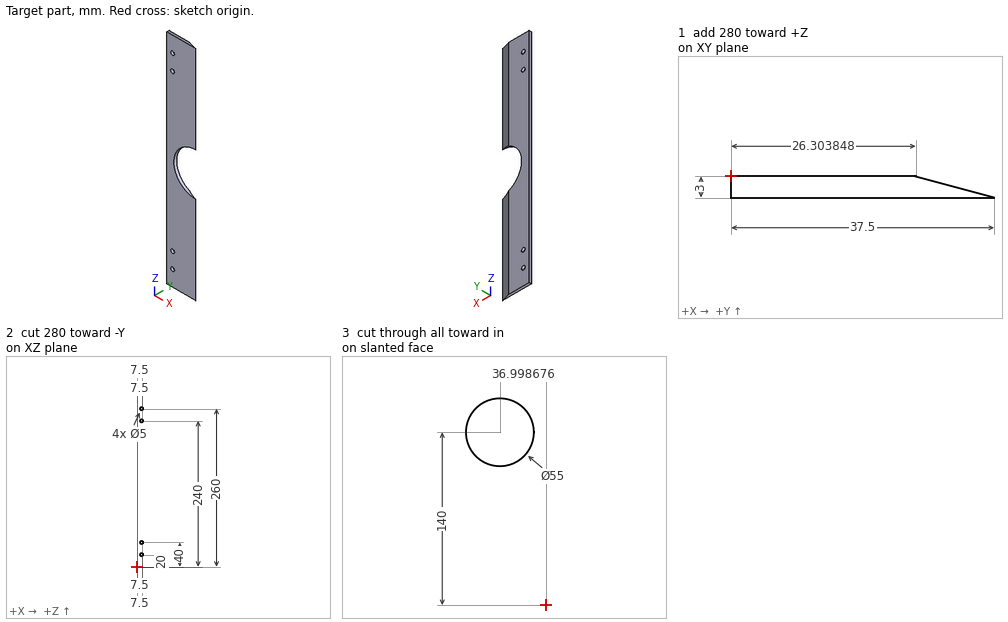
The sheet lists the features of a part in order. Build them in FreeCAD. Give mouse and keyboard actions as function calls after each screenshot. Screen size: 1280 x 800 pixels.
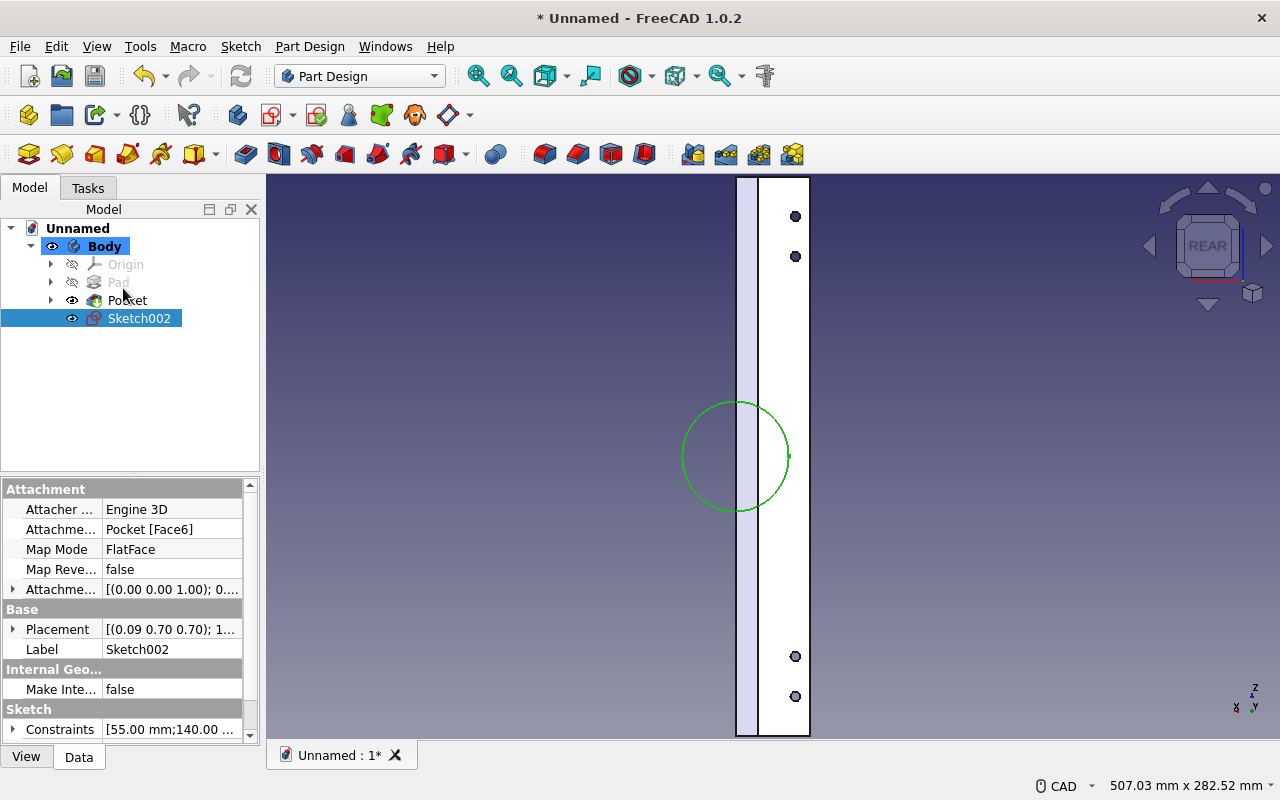
click(246, 154)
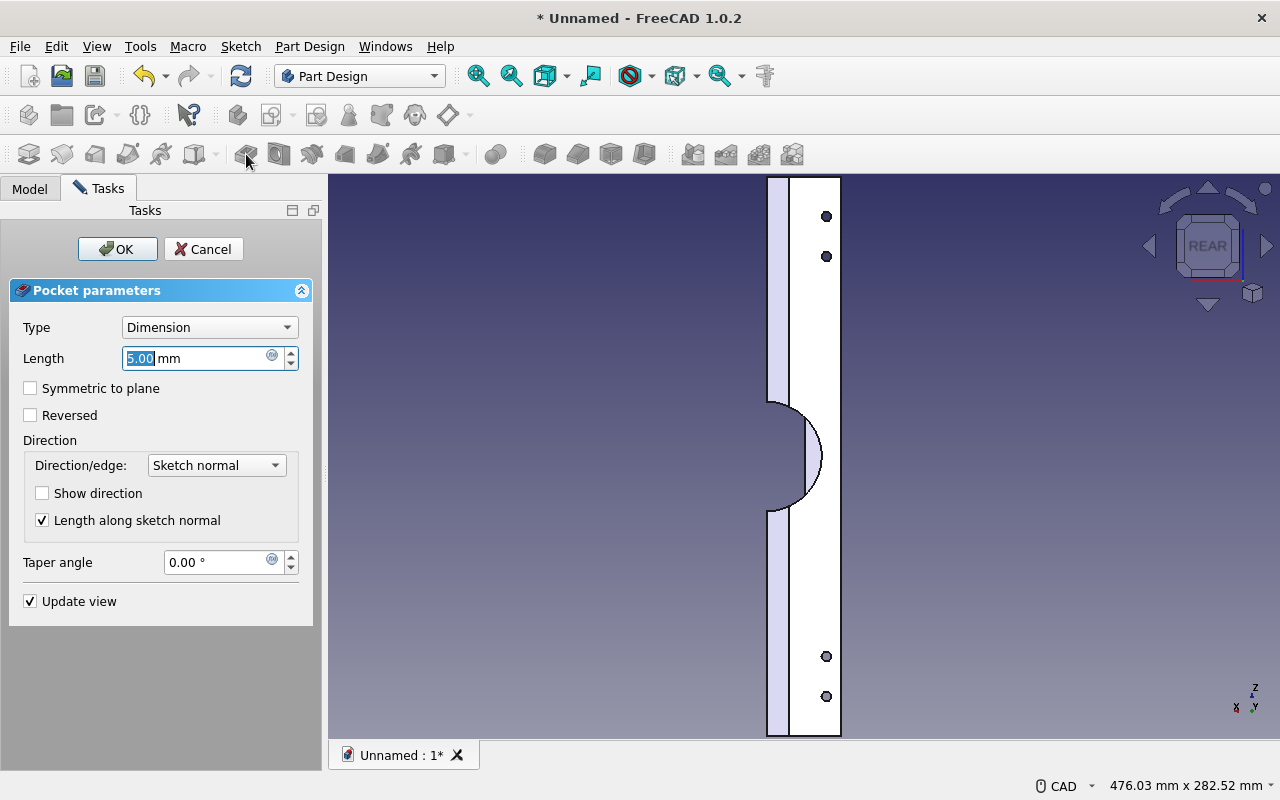
click(210, 328)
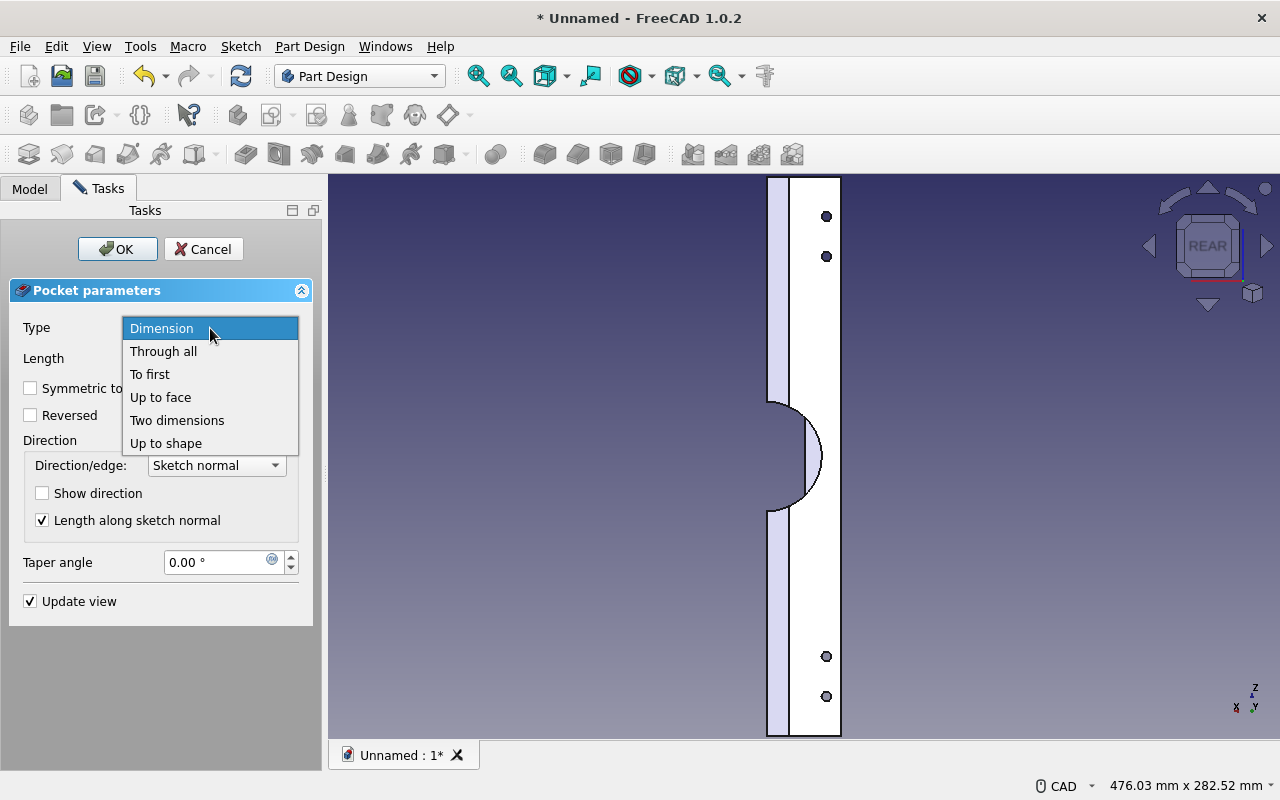
click(208, 352)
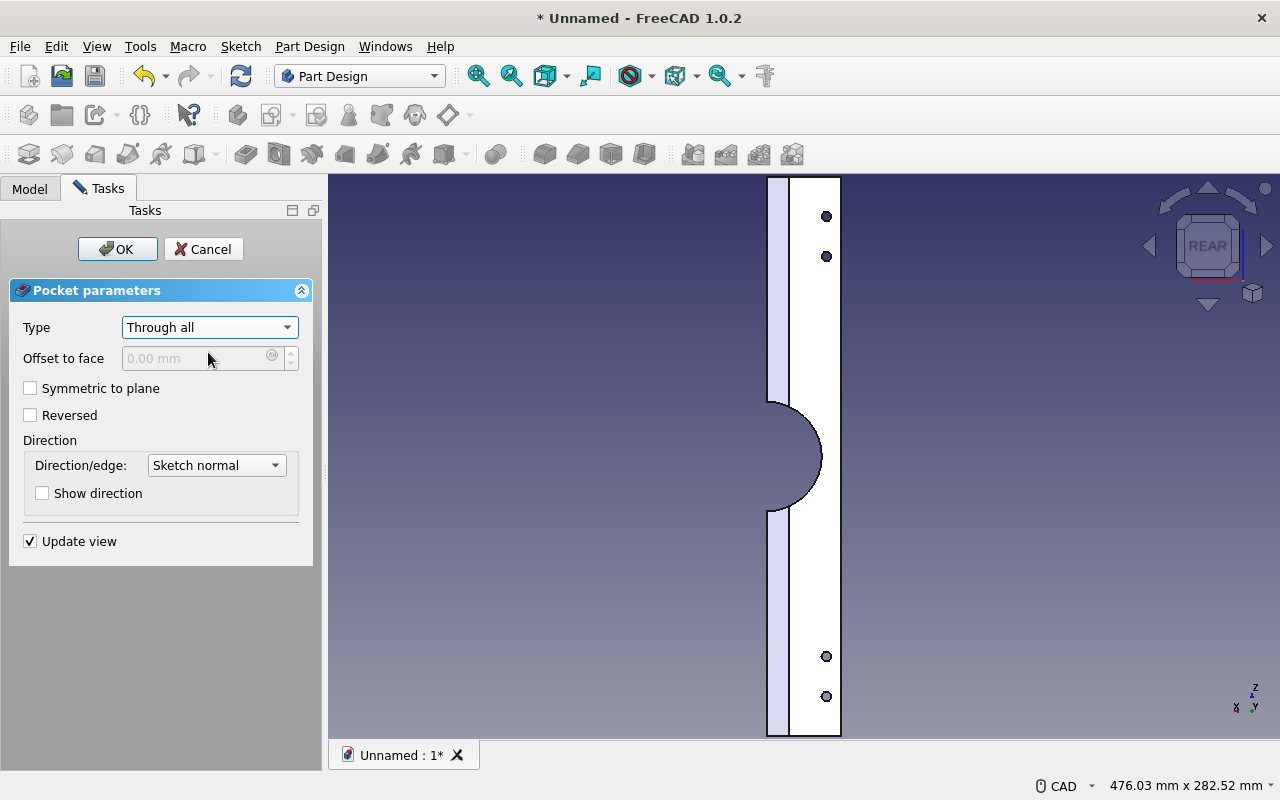
click(118, 249)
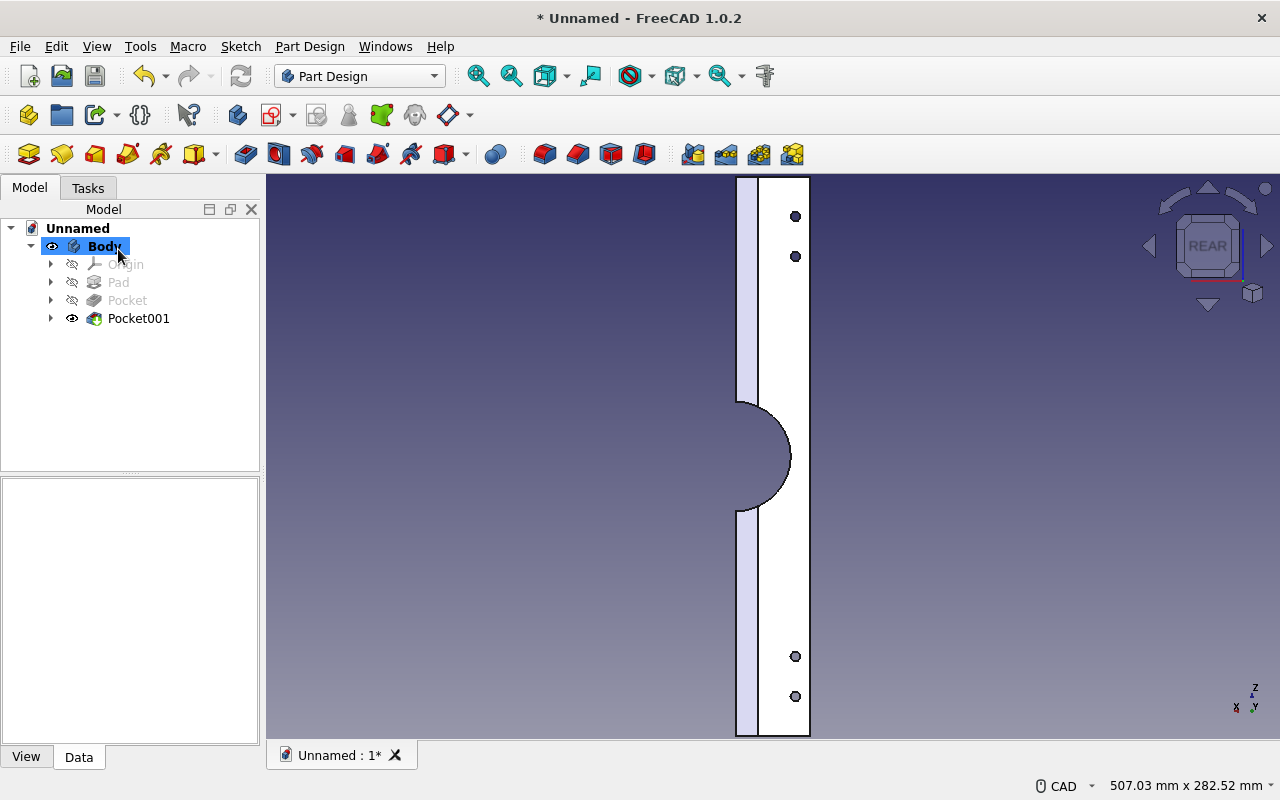
key(0)